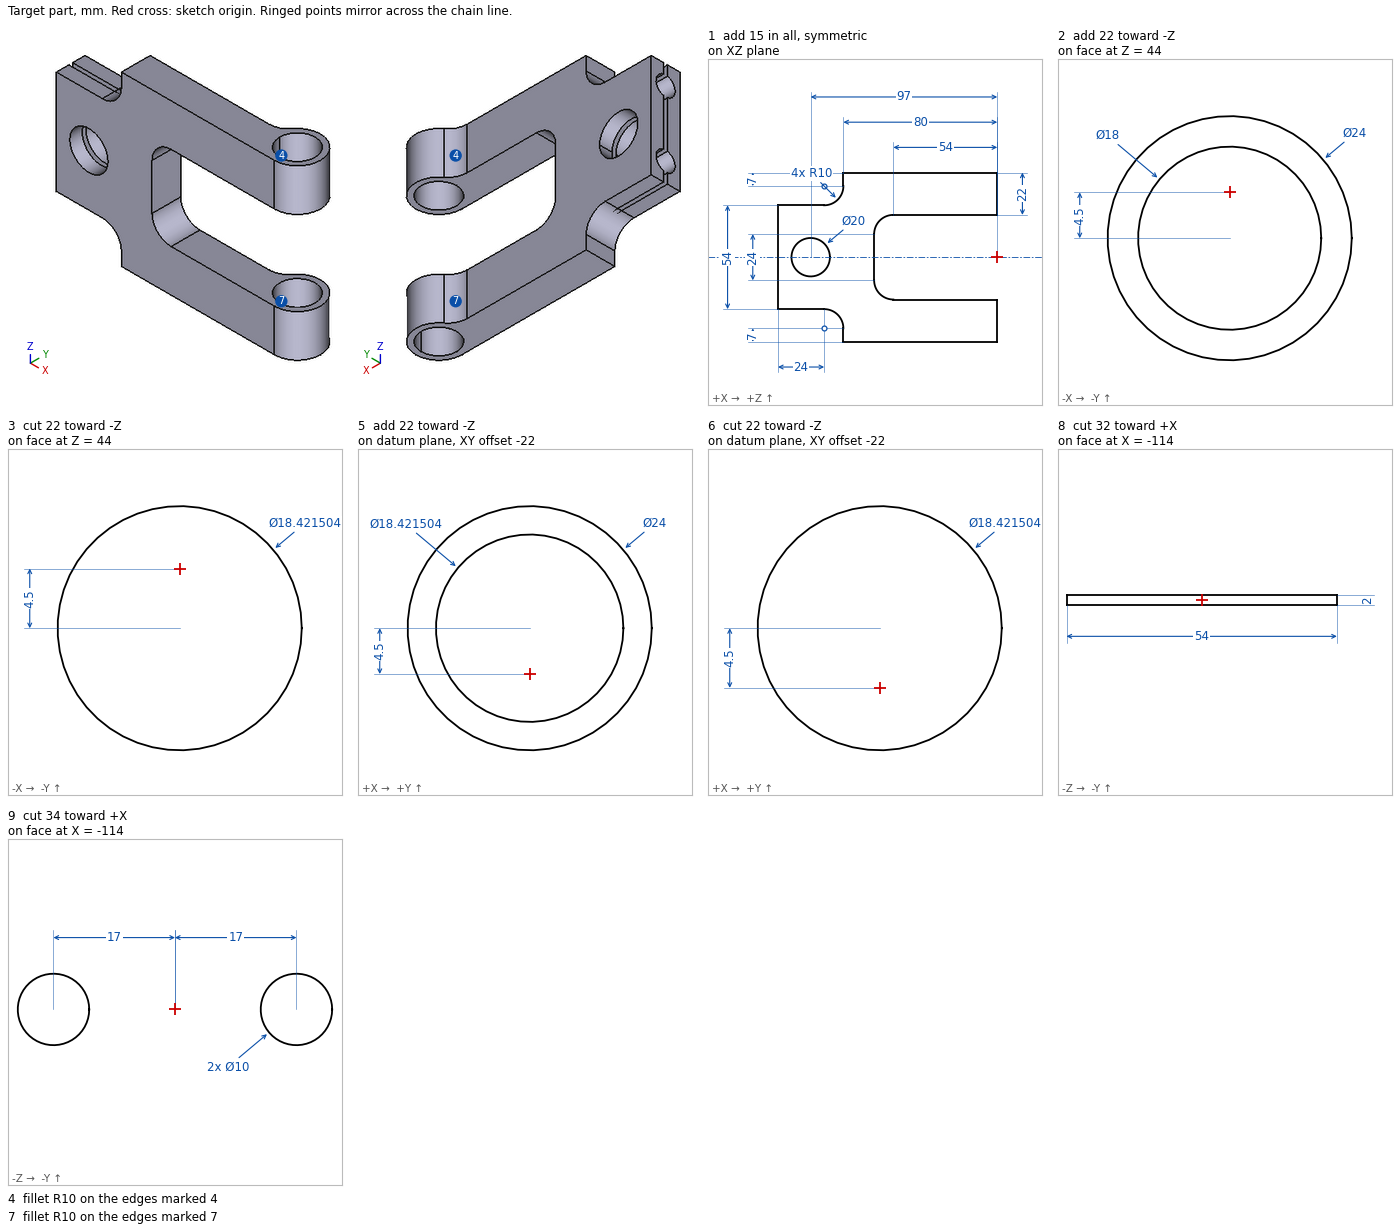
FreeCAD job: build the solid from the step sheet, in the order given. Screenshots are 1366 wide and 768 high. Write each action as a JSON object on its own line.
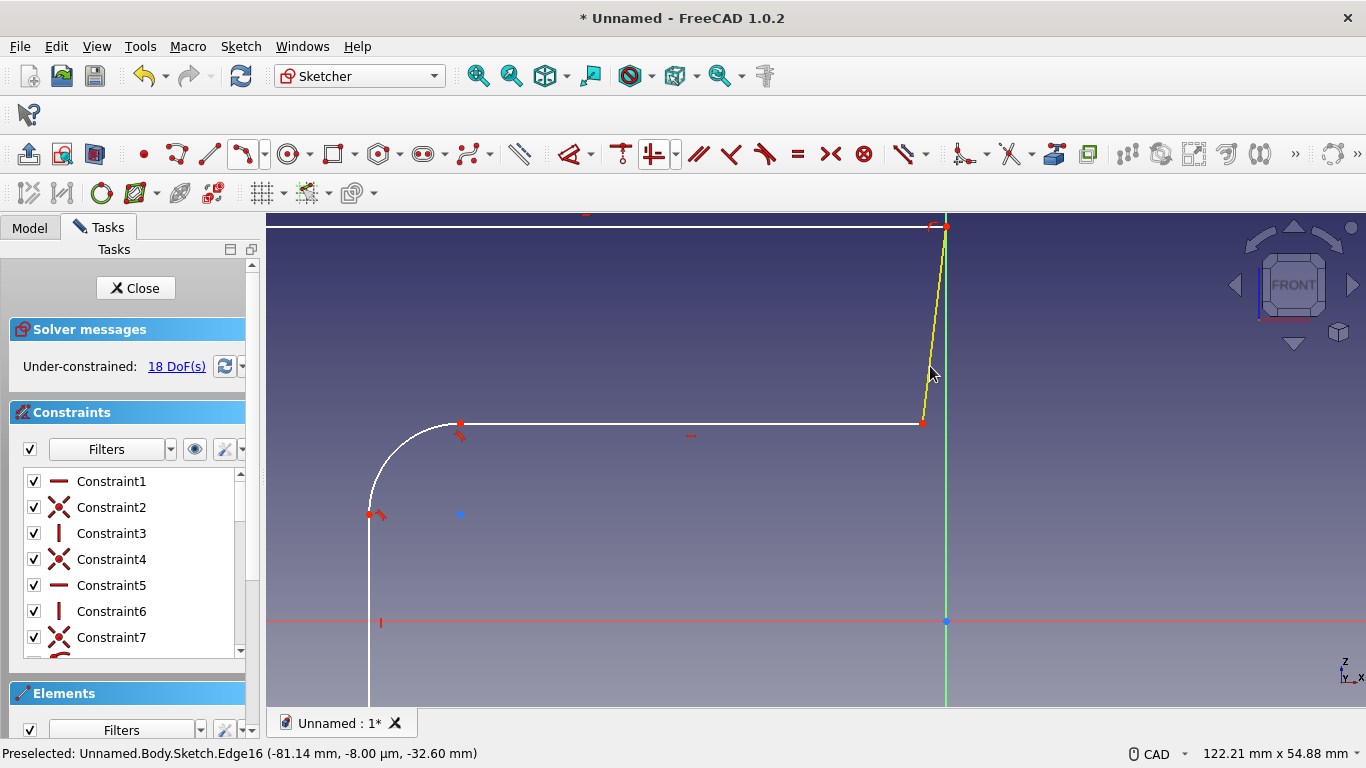
{"action": "left_click", "coordinate": [930, 365]}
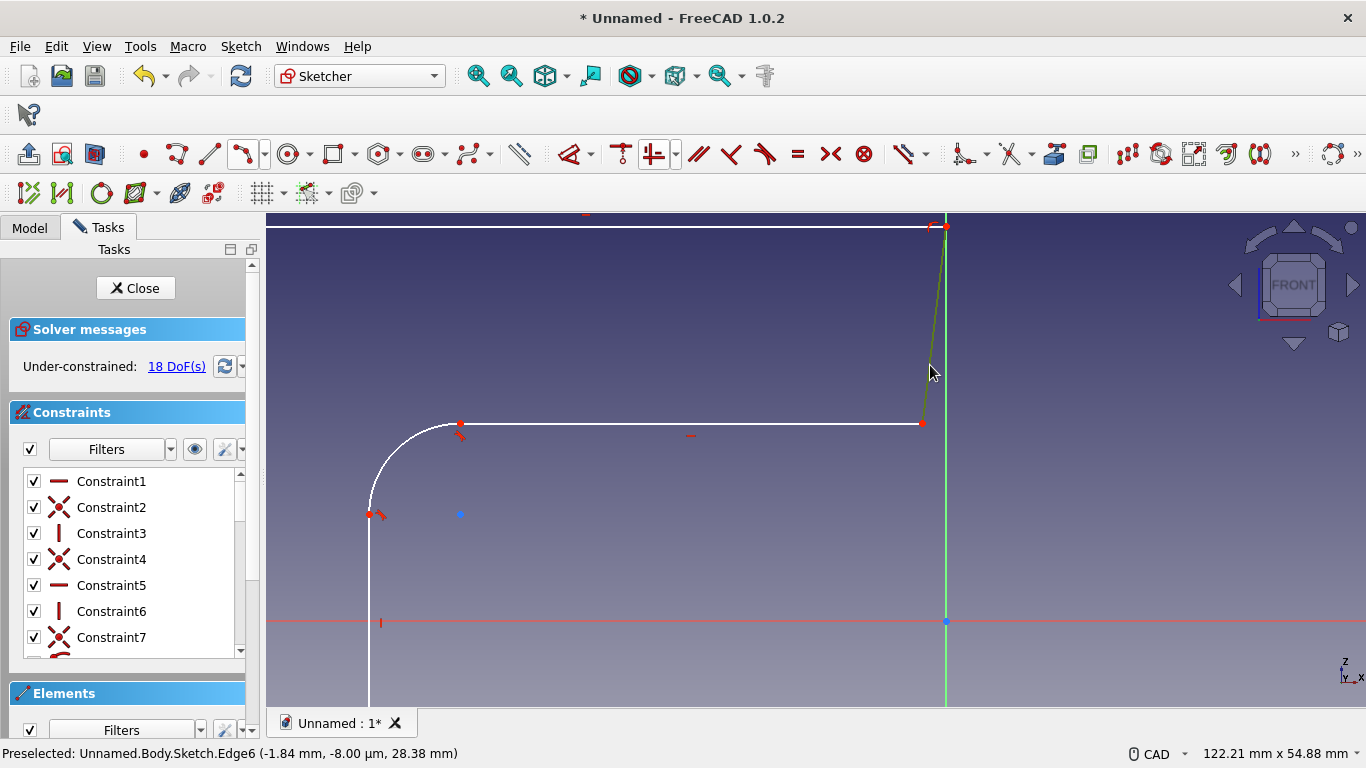
{"action": "key", "text": "v"}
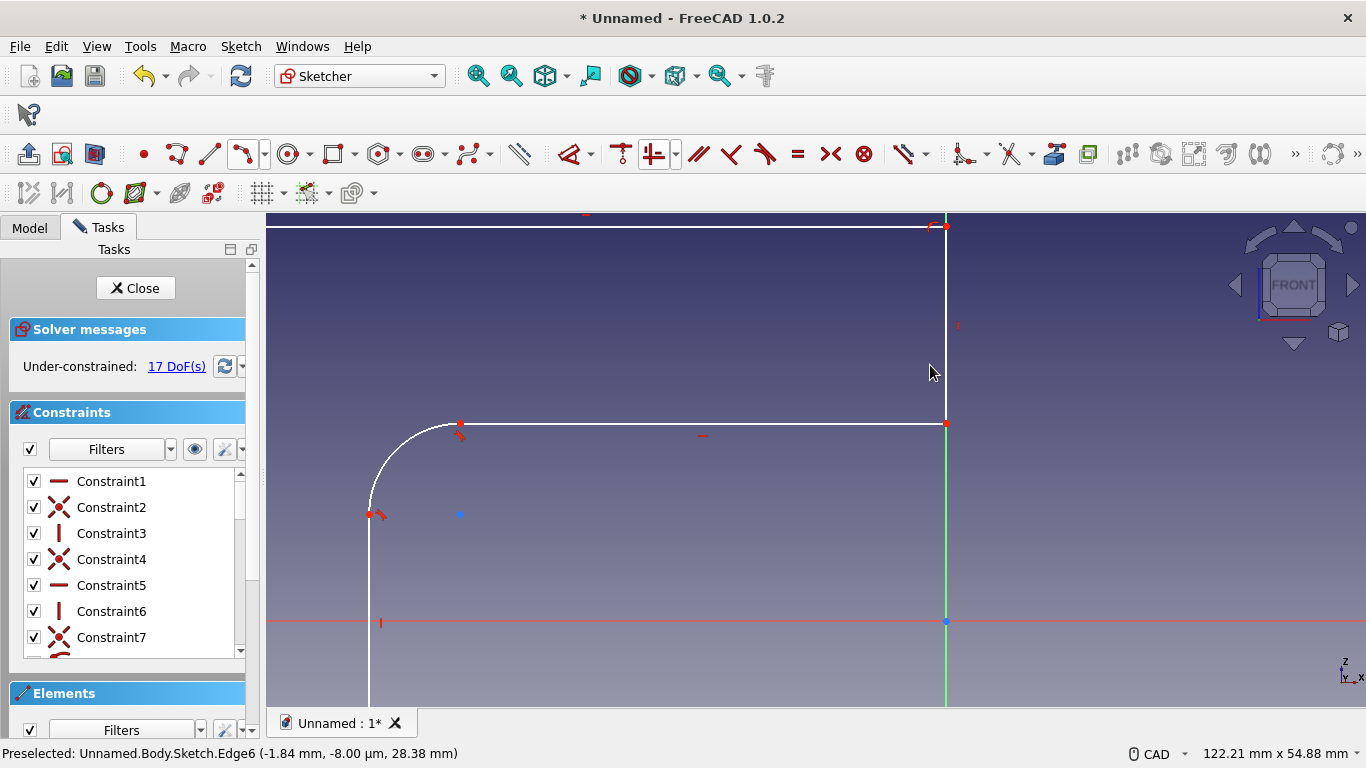
{"action": "scroll", "coordinate": [931, 366], "scroll_direction": "down", "scroll_amount": 5}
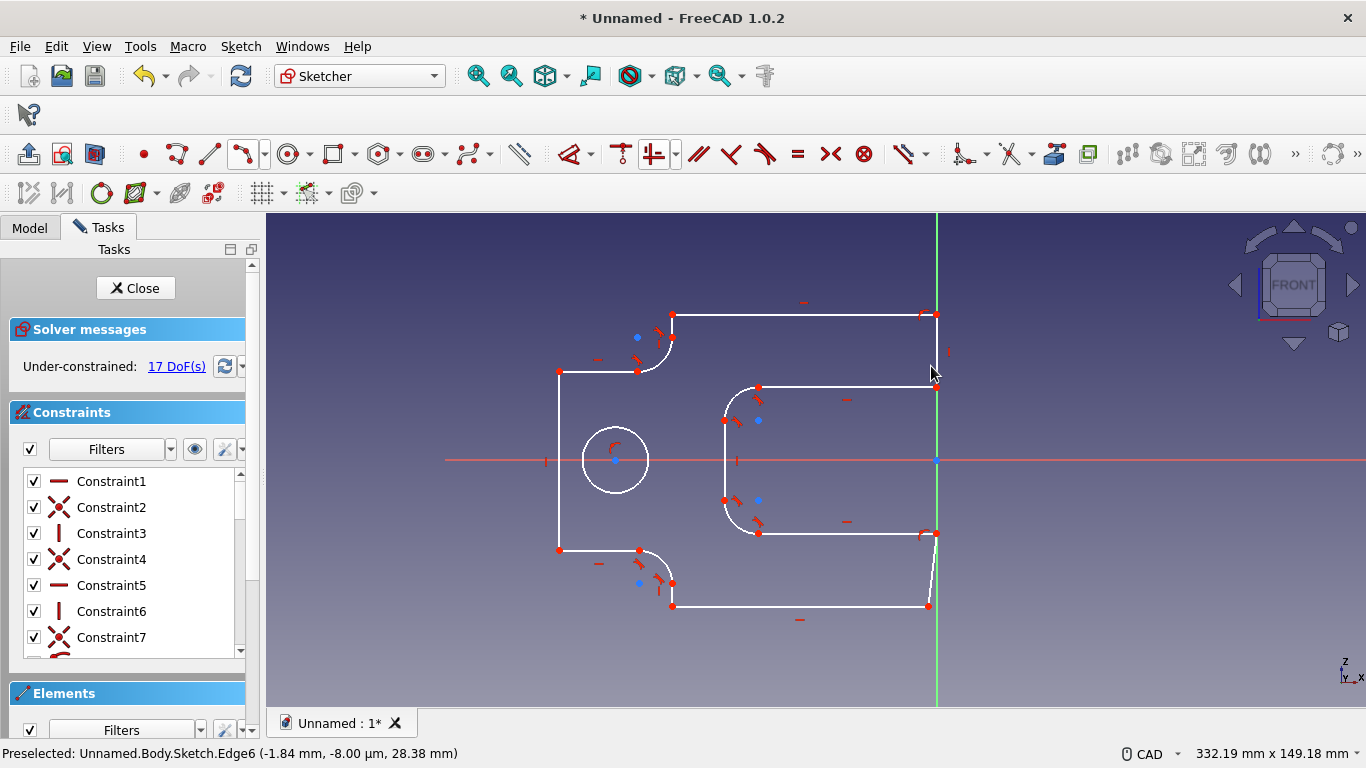
{"action": "scroll", "coordinate": [931, 585], "scroll_direction": "up", "scroll_amount": 5}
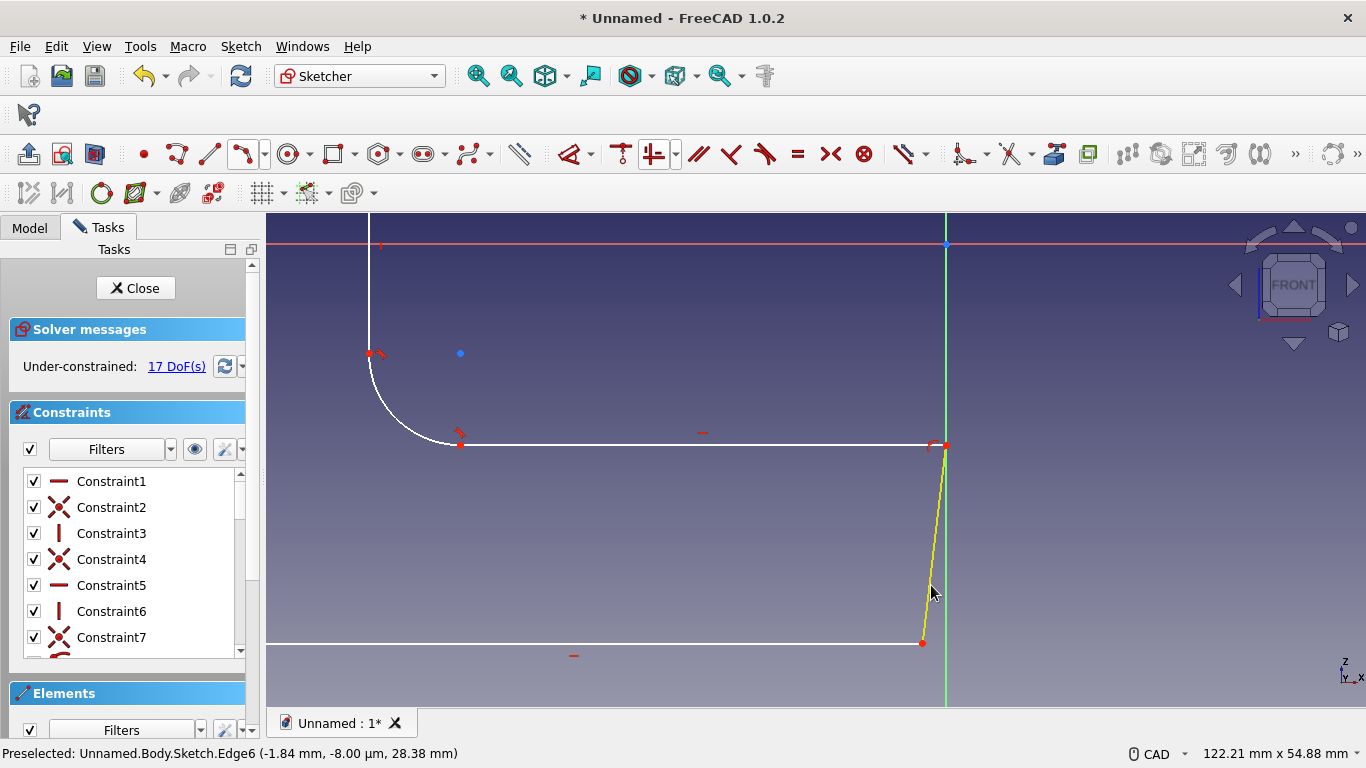
{"action": "left_click", "coordinate": [930, 584]}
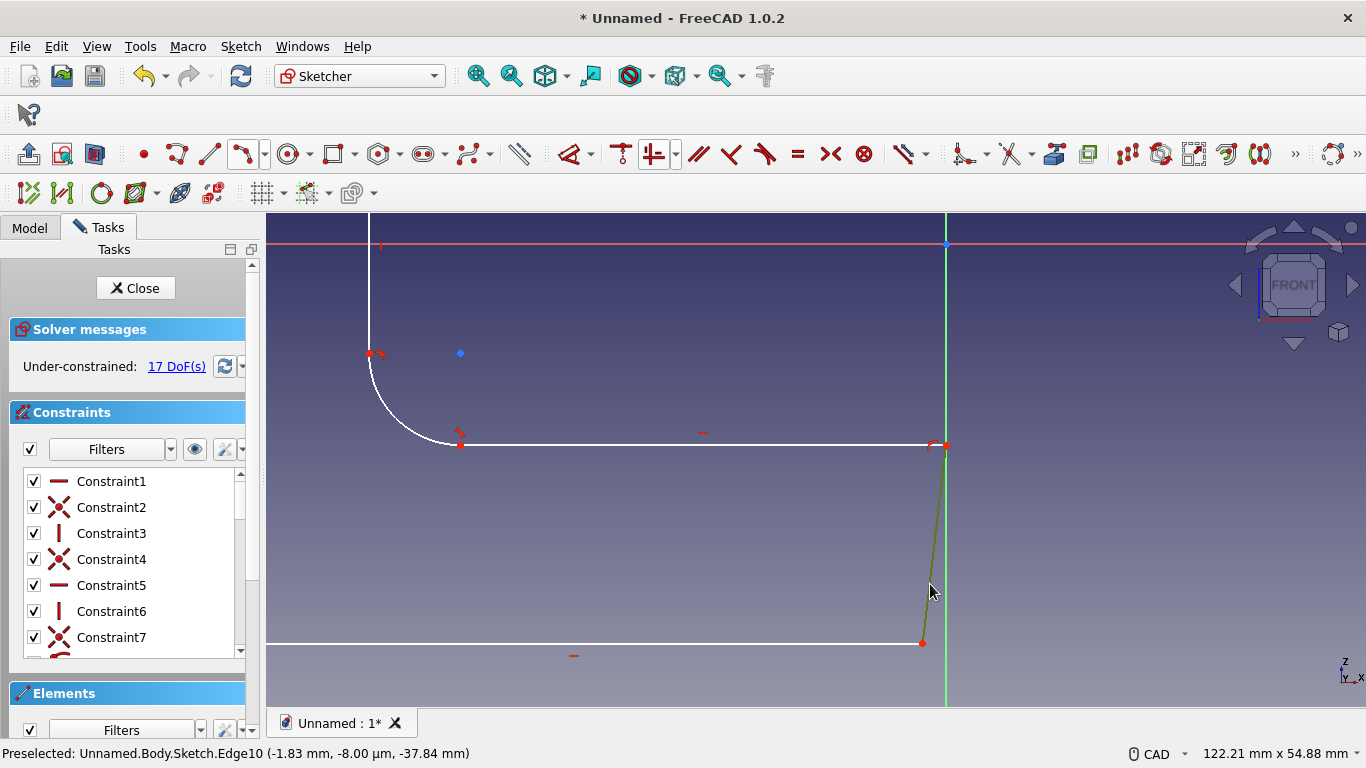
{"action": "left_click", "coordinate": [676, 154]}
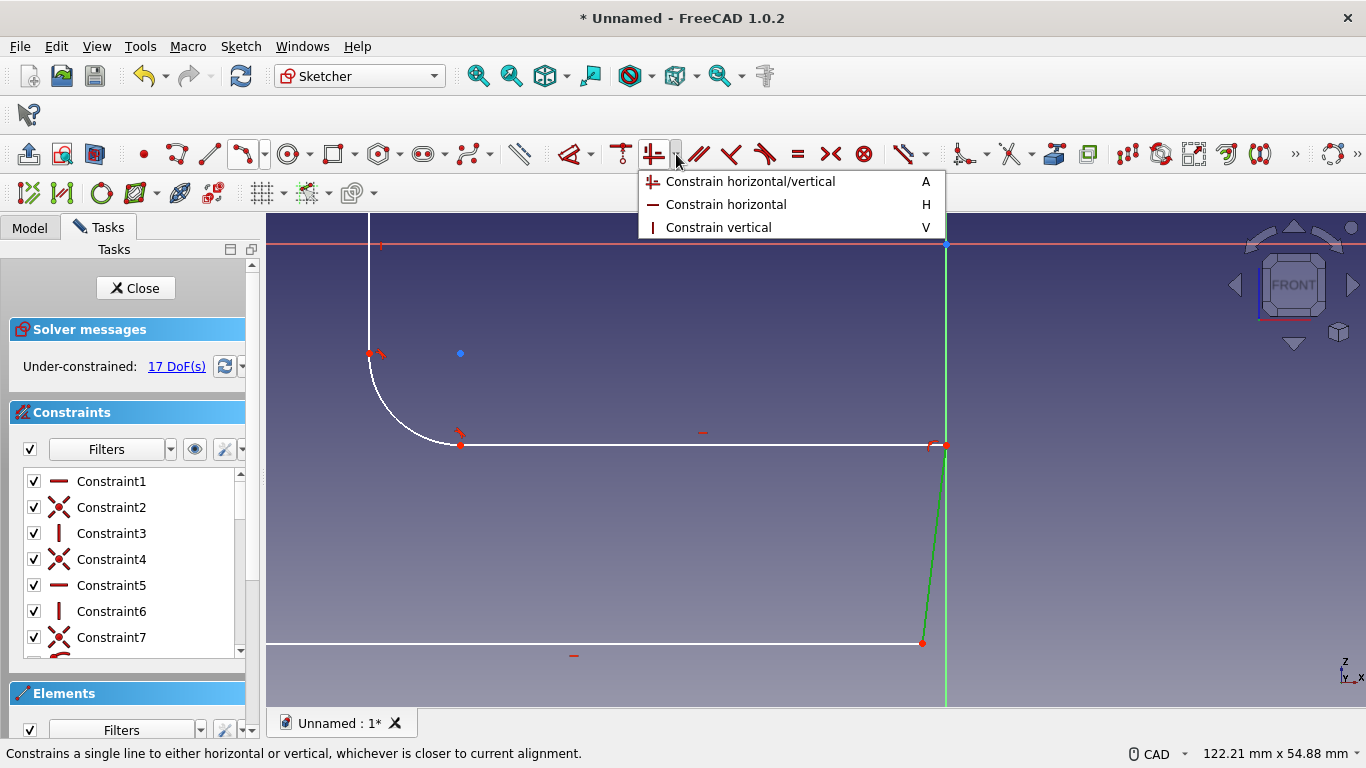
{"action": "left_click", "coordinate": [792, 228]}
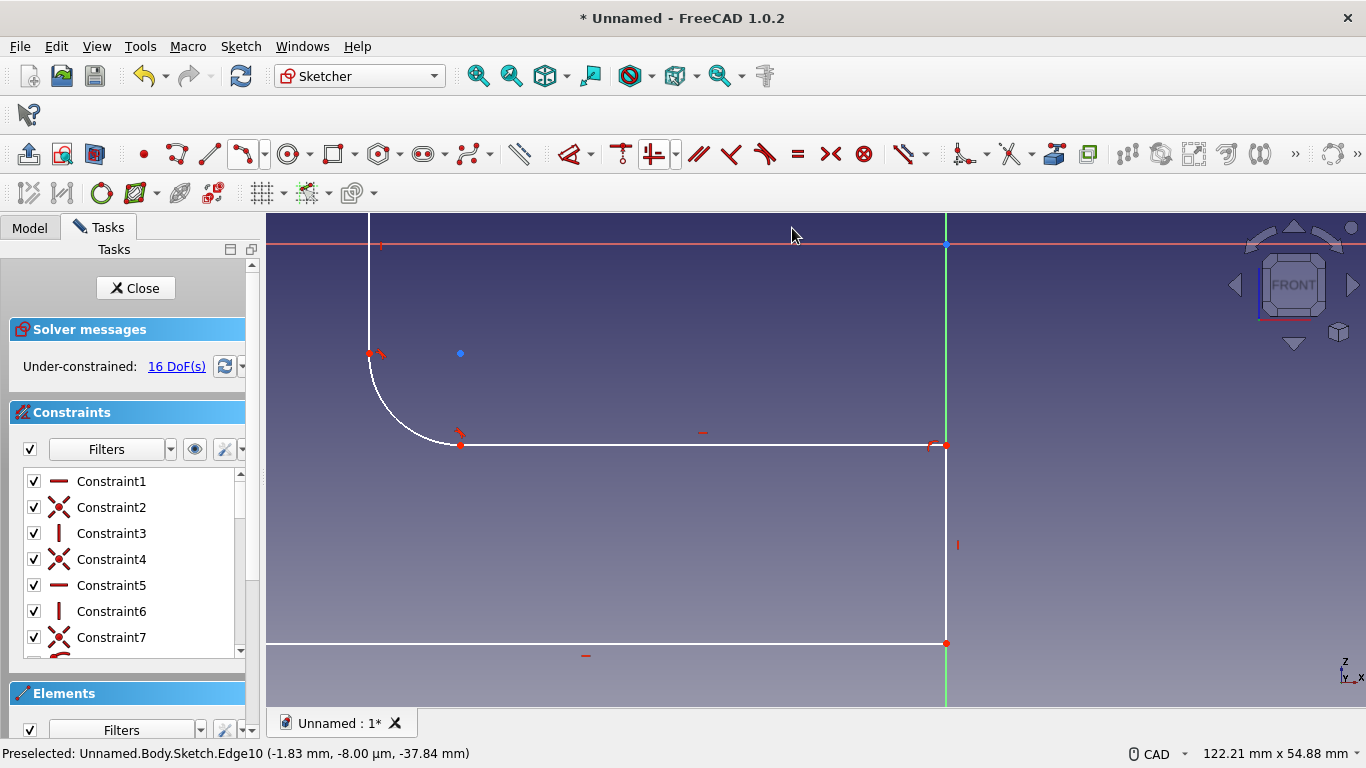
{"action": "scroll", "coordinate": [931, 585], "scroll_direction": "down", "scroll_amount": 5}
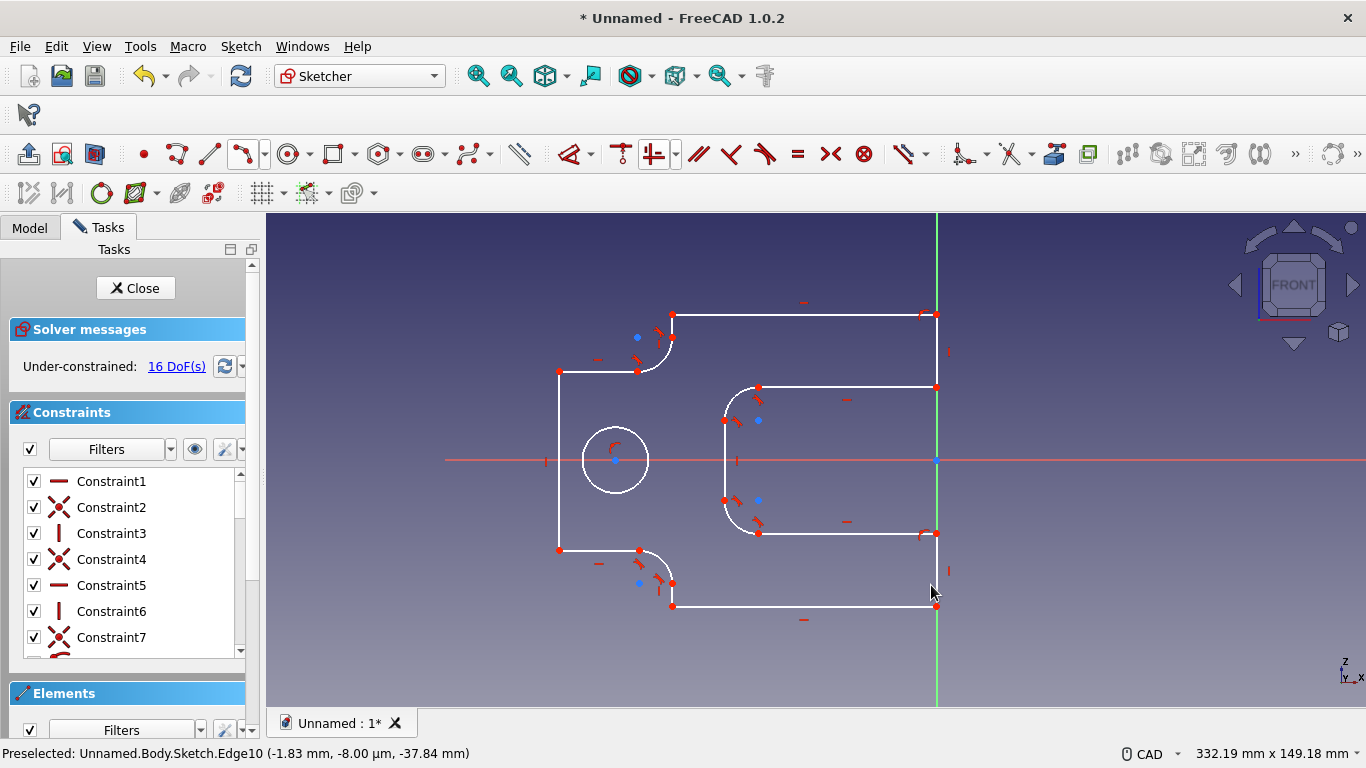
{"action": "left_click", "coordinate": [653, 368]}